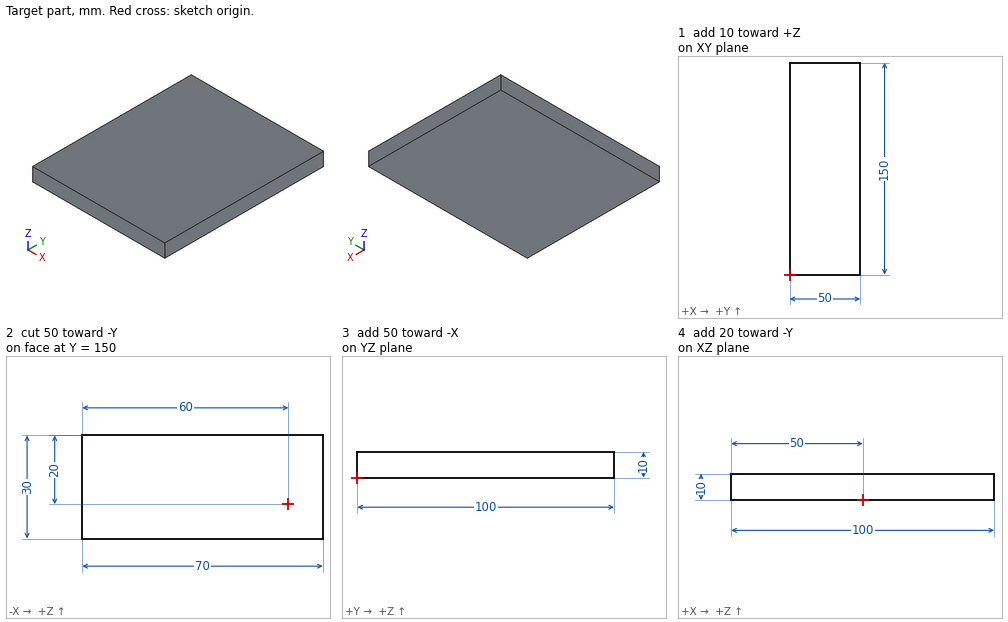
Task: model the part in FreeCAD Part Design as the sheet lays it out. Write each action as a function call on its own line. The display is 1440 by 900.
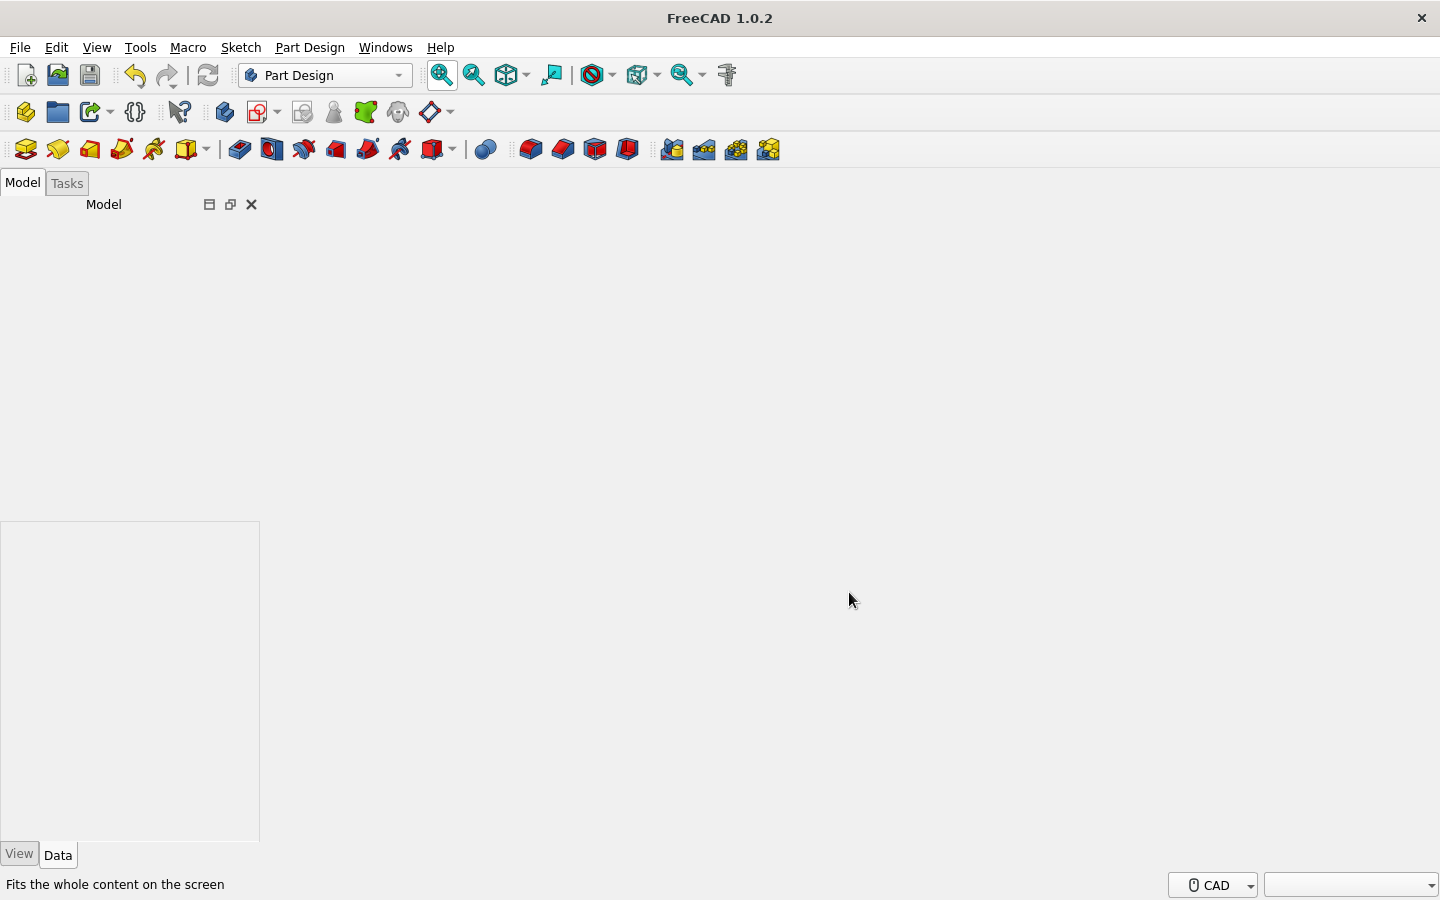
click(26, 76)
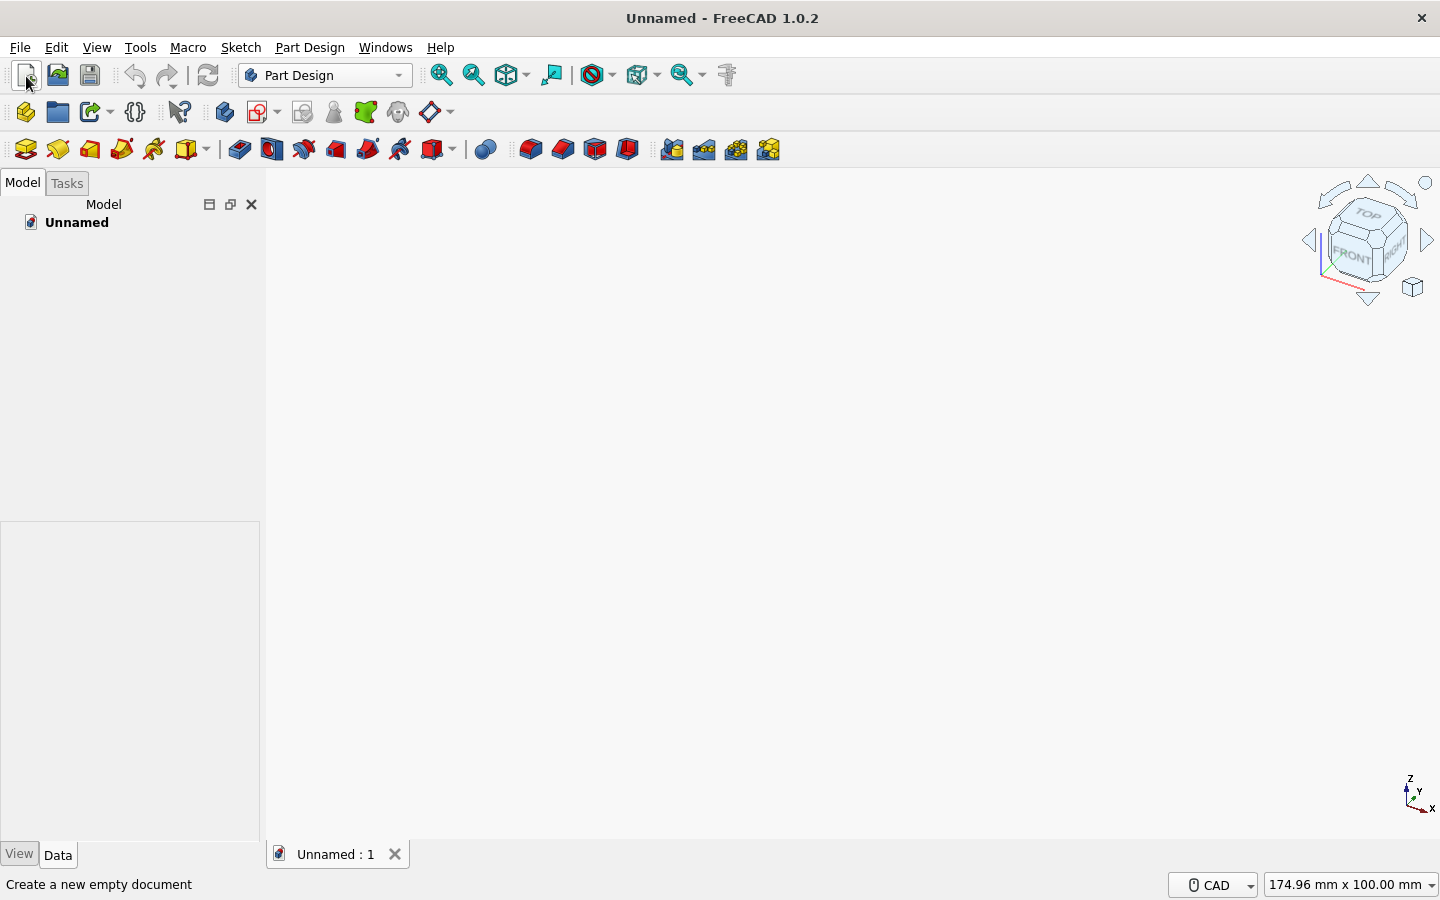
click(258, 112)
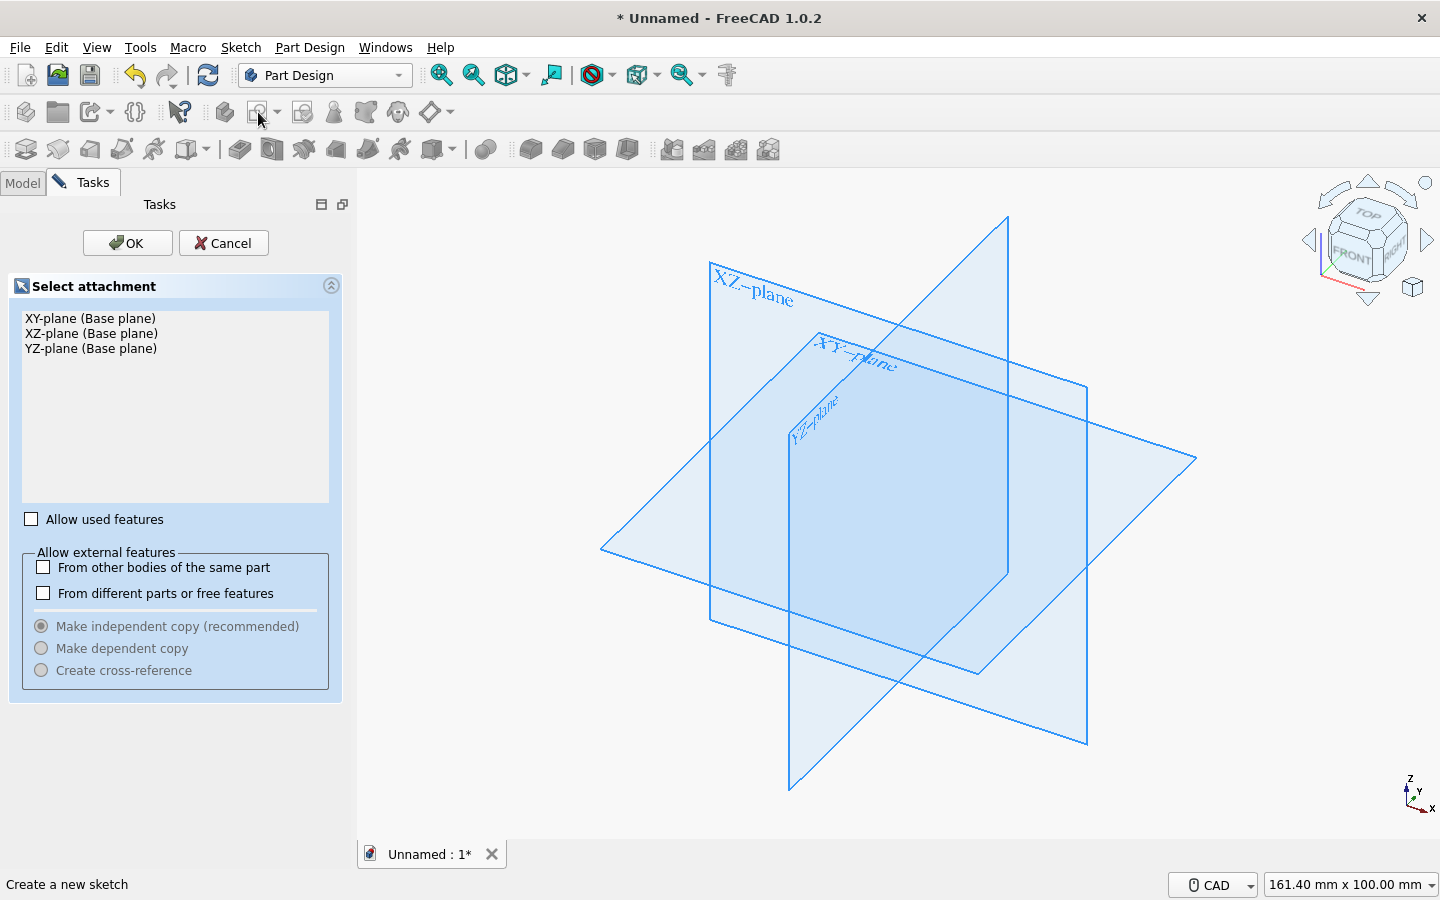
click(82, 318)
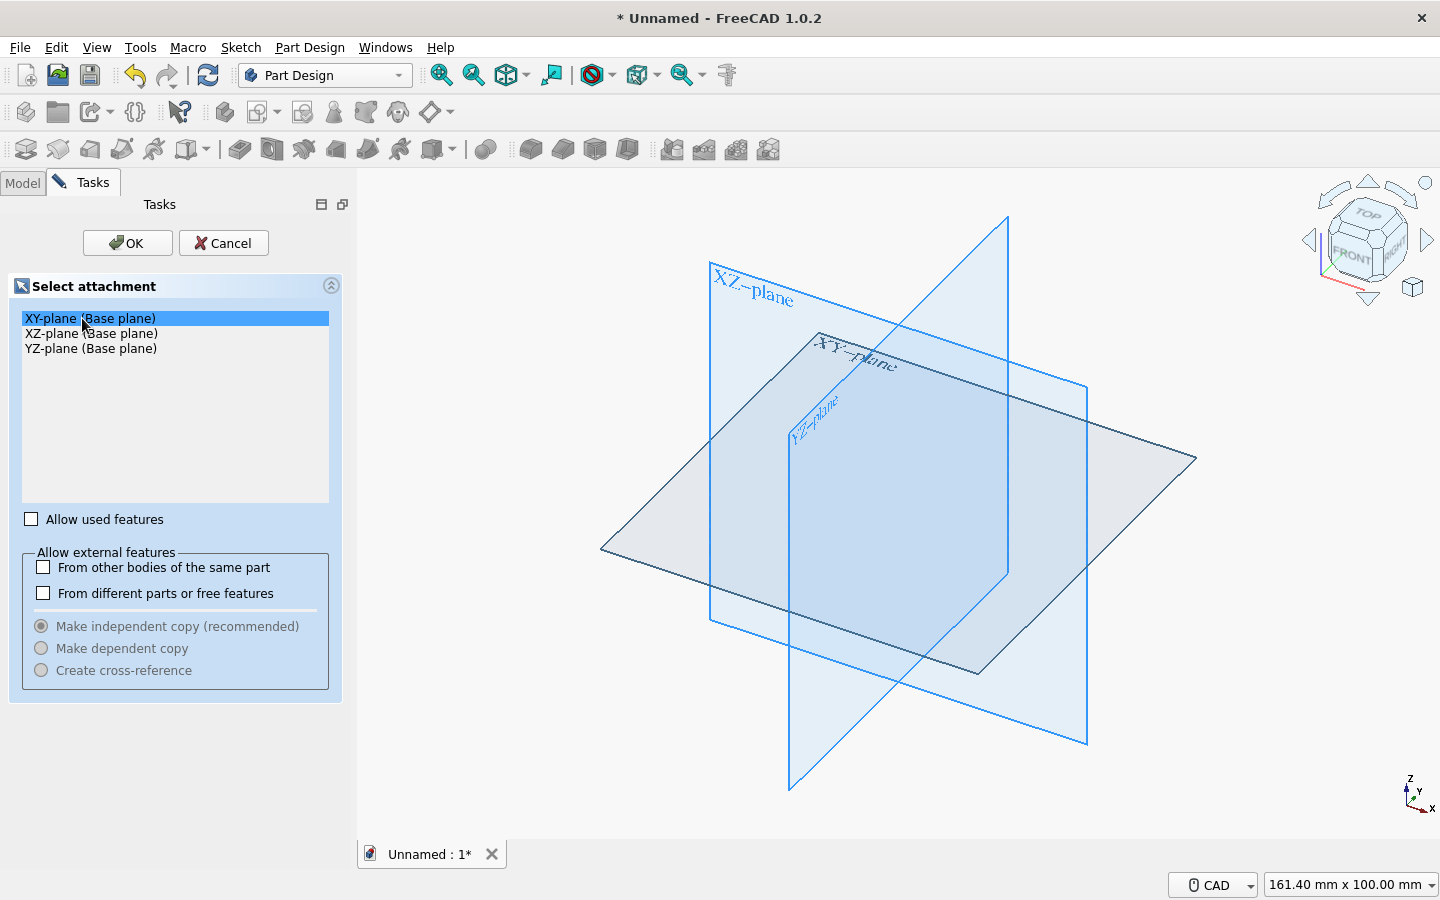
click(128, 243)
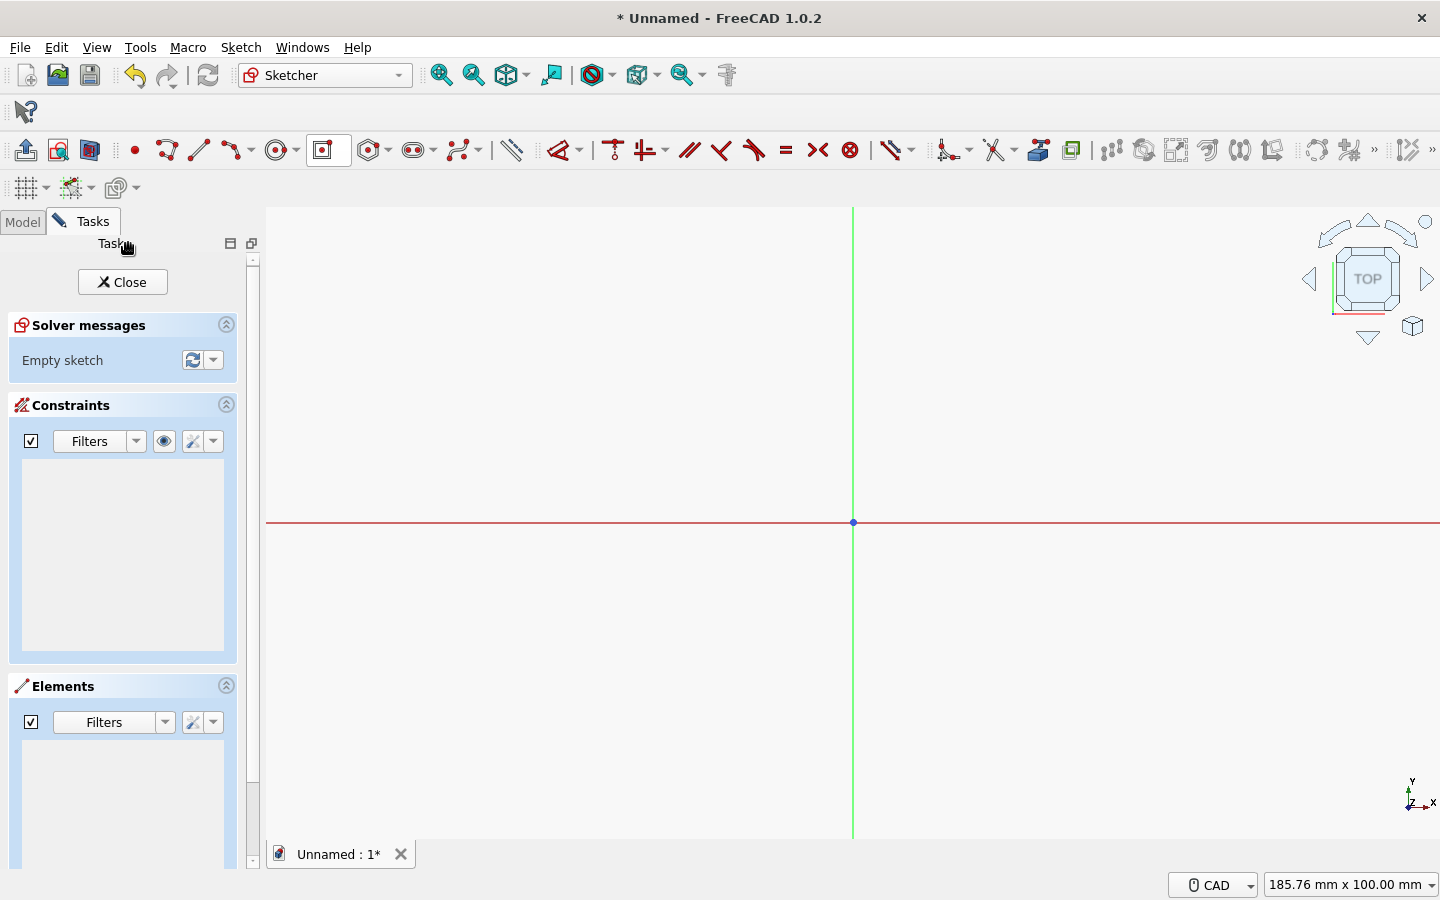
scroll(653, 799, down, 5)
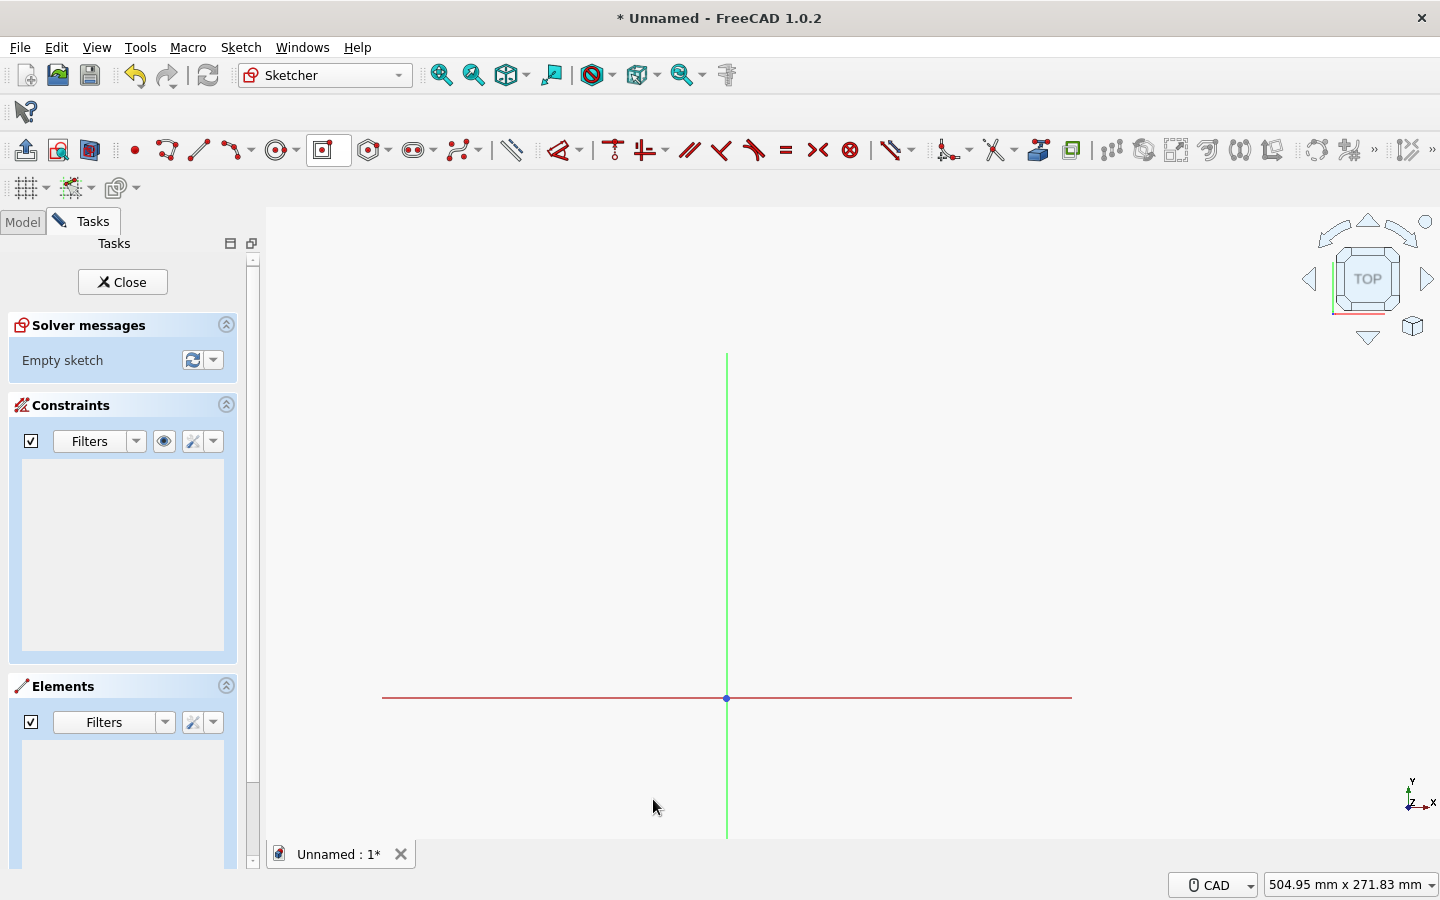
click(346, 150)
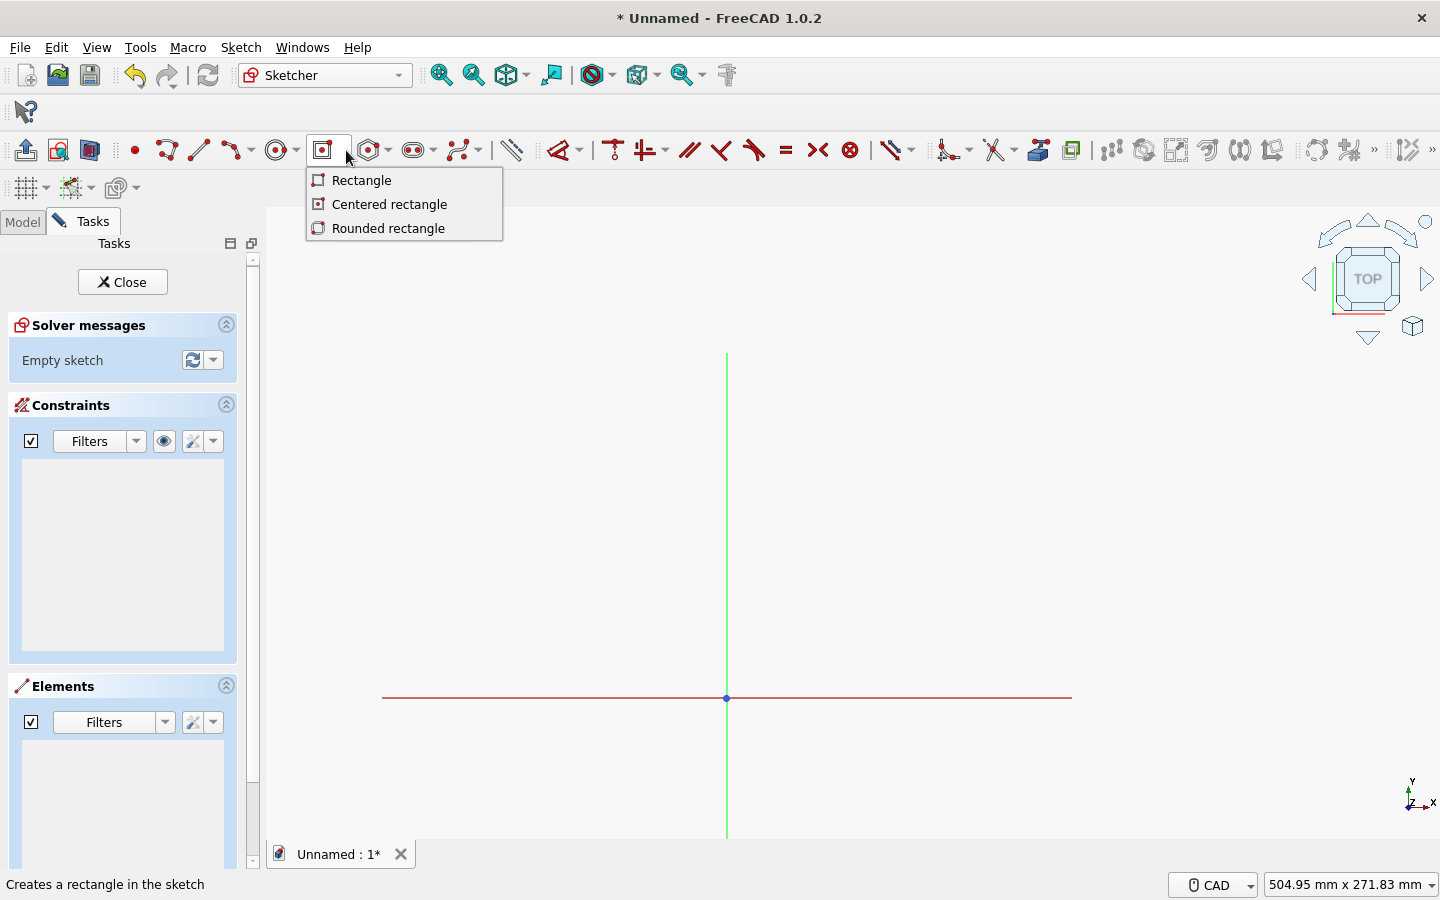
click(404, 180)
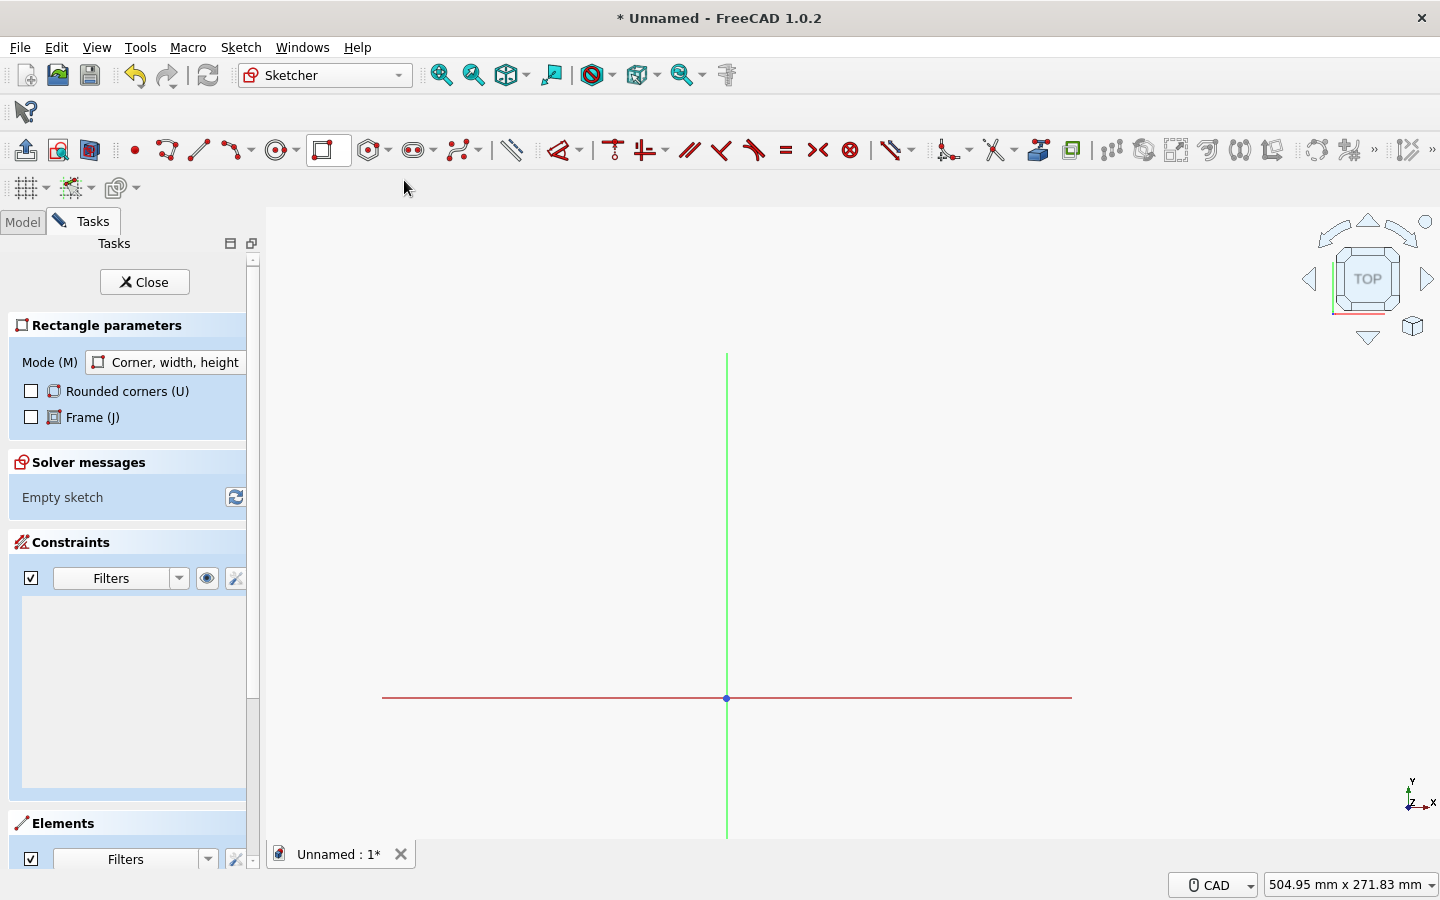
click(727, 698)
click(843, 349)
key(Escape)